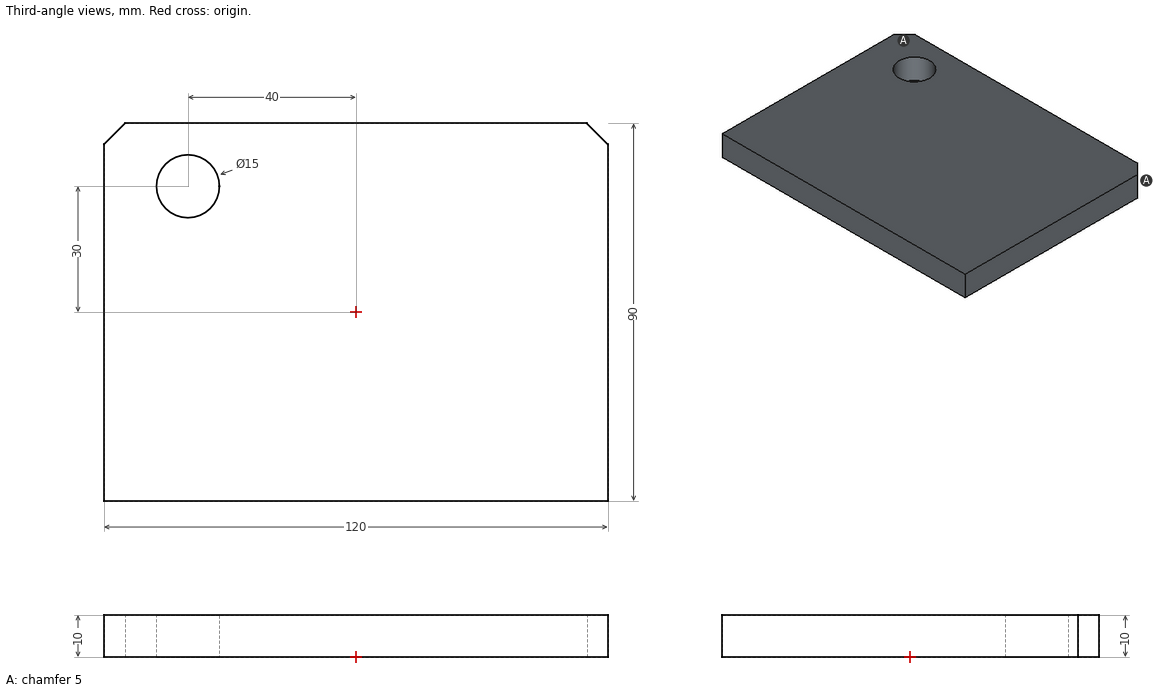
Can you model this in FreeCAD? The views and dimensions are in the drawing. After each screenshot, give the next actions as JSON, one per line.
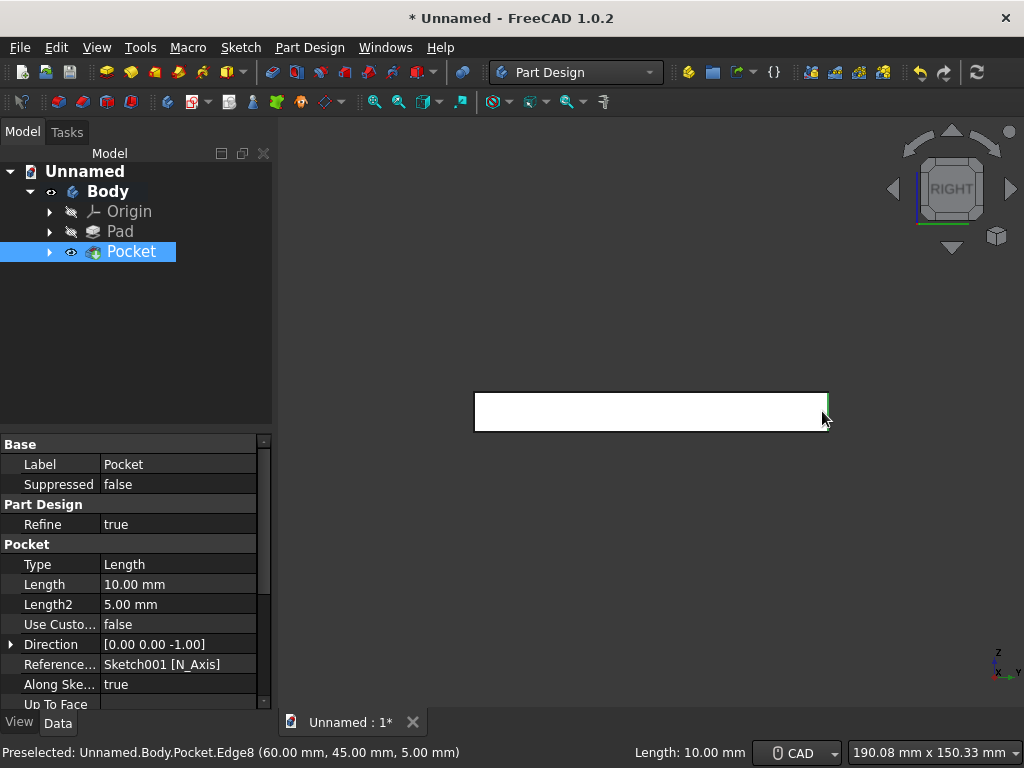
{"action": "key", "text": "5"}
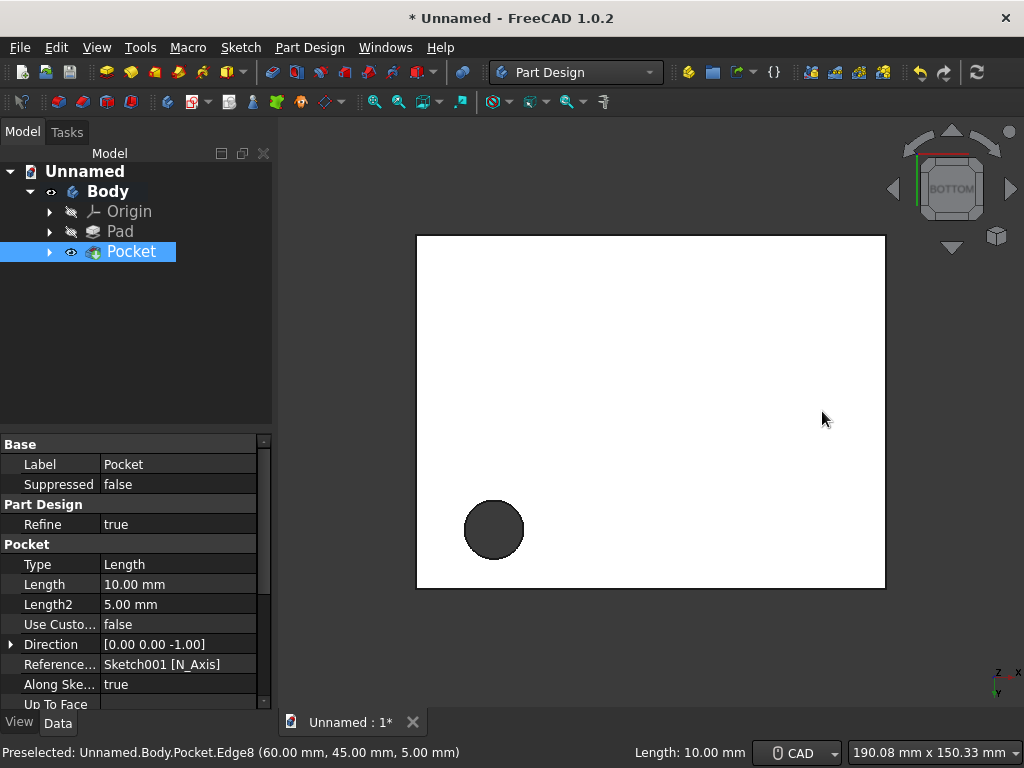
{"action": "key", "text": "4"}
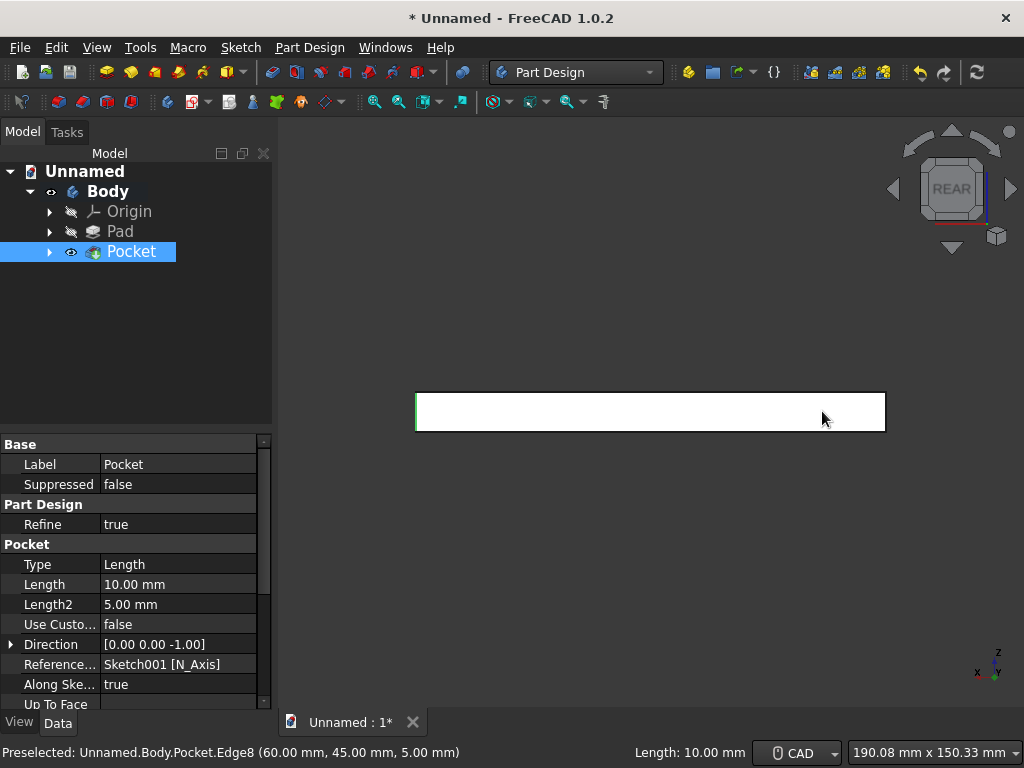
{"action": "left_click", "coordinate": [886, 411], "text": "ctrl"}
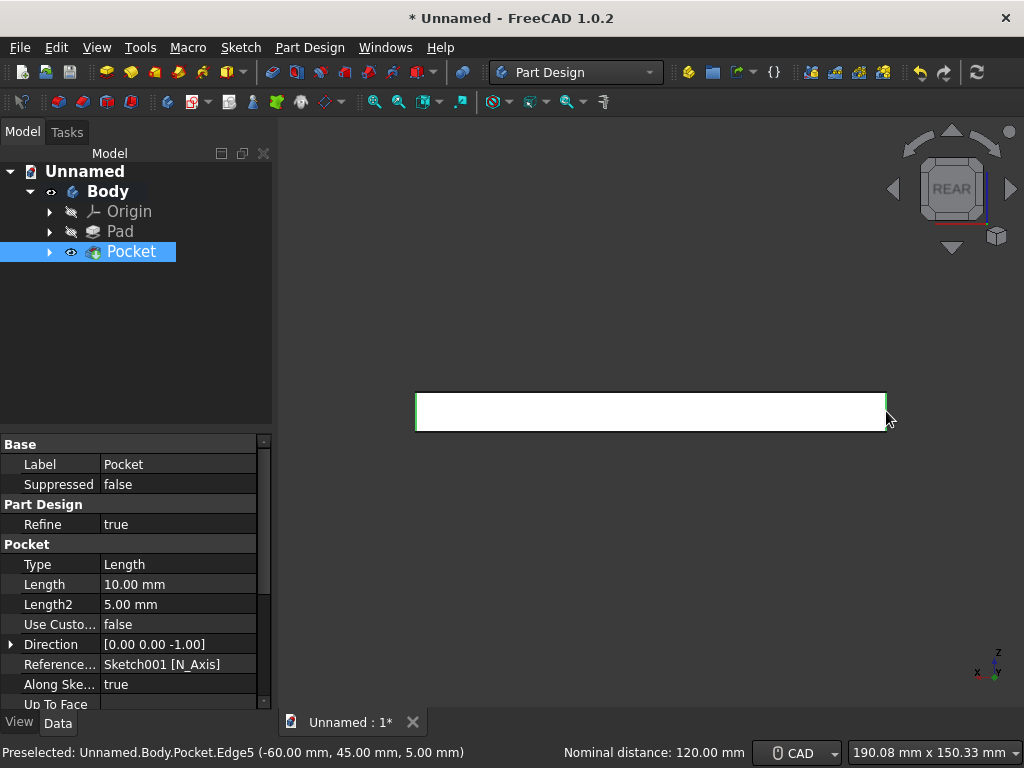
{"action": "left_click", "coordinate": [84, 102]}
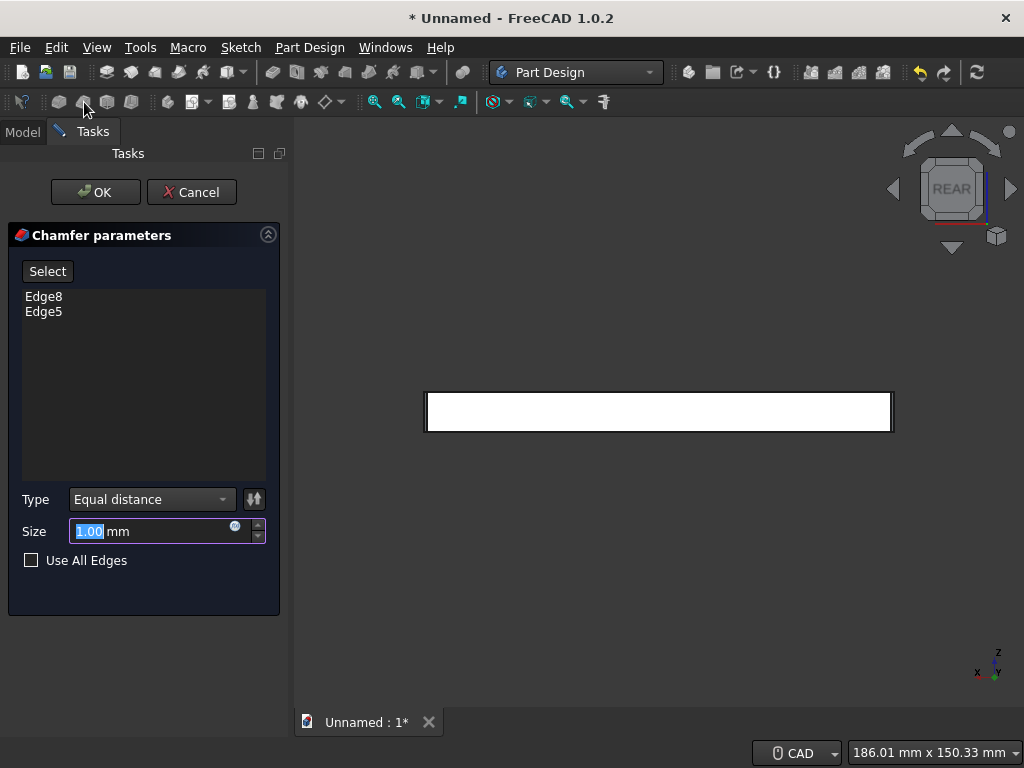
{"action": "type", "text": "5"}
{"action": "key", "text": "Tab"}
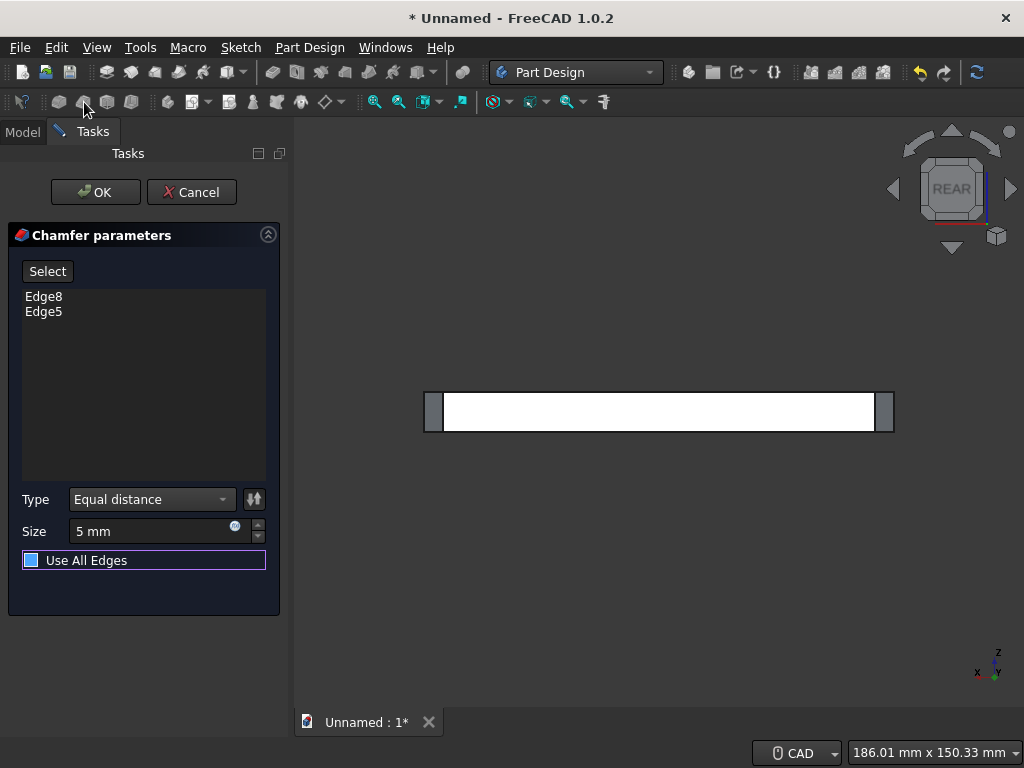
{"action": "left_click", "coordinate": [96, 192]}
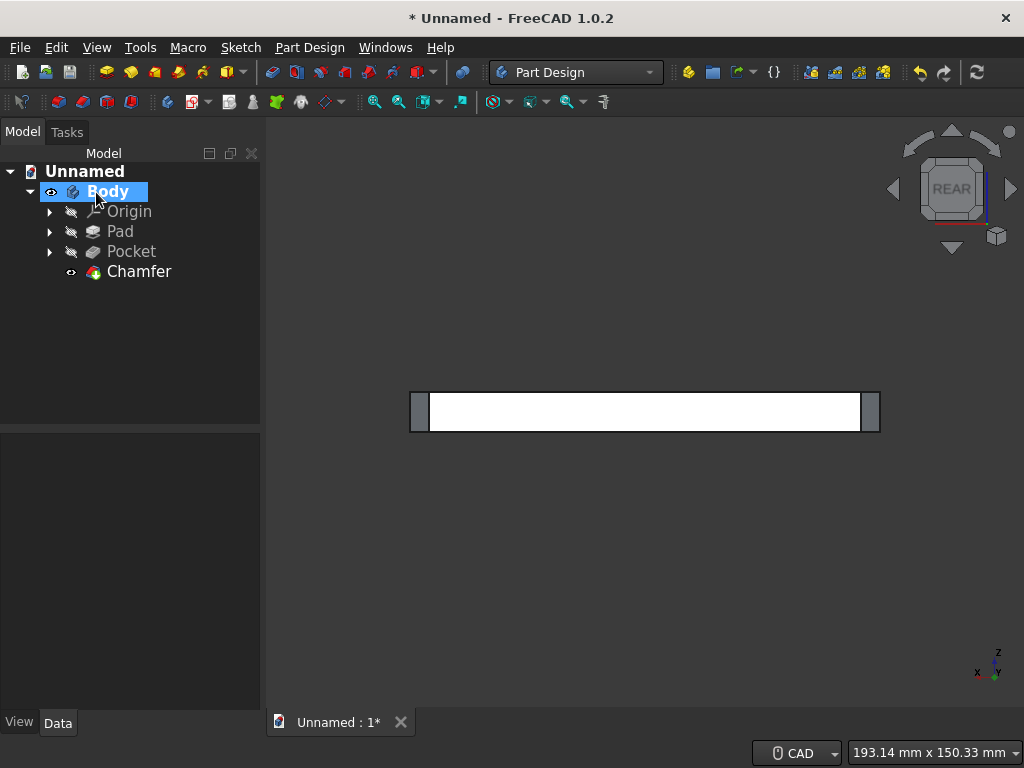
{"action": "key", "text": "0"}